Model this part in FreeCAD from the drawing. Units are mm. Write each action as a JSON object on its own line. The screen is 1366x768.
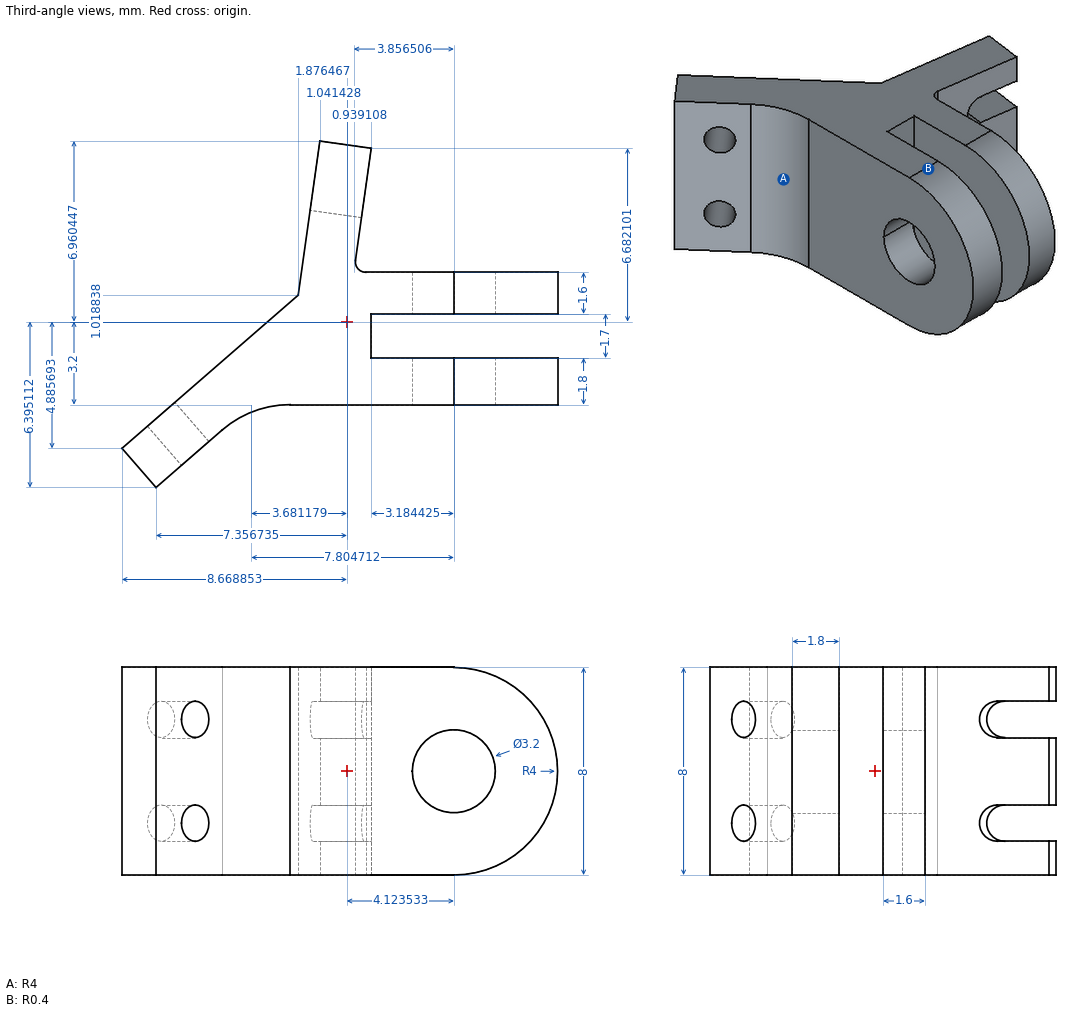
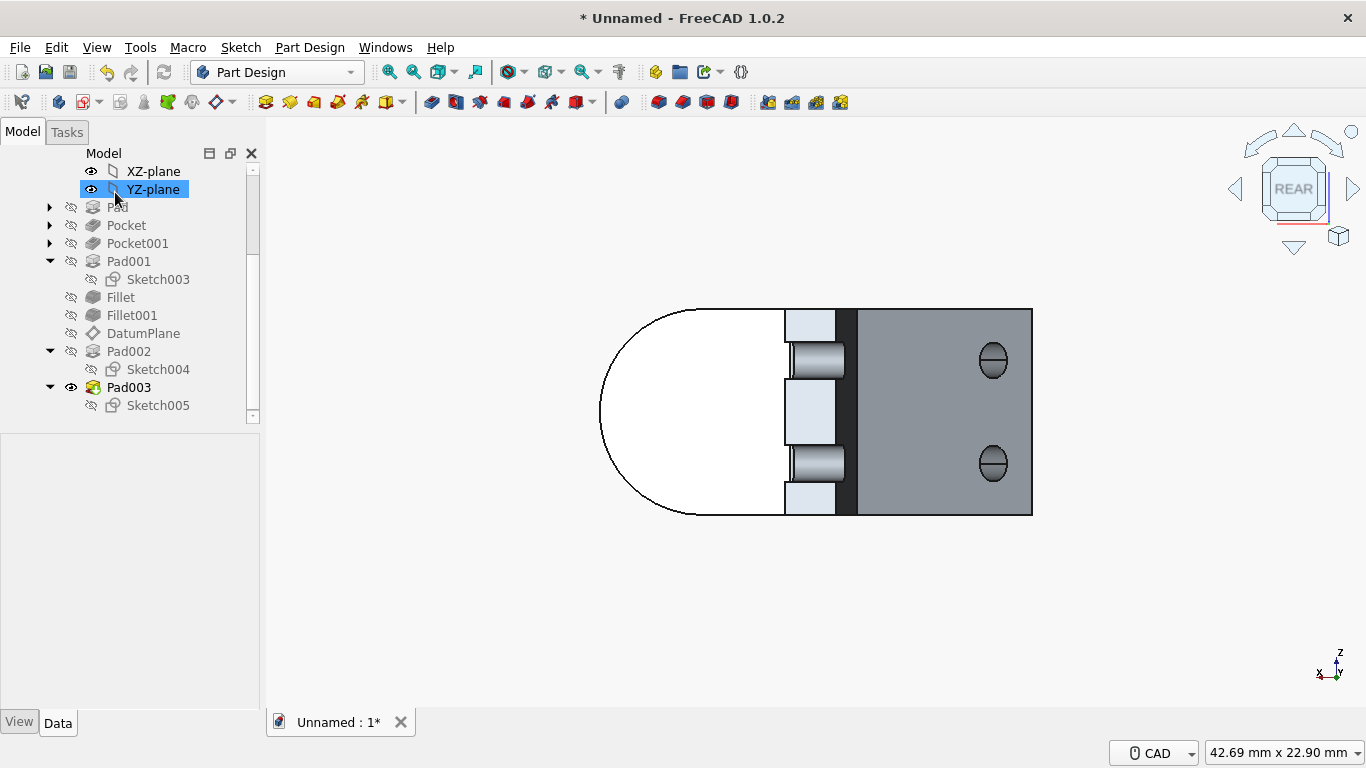
{"action": "left_click", "coordinate": [390, 72]}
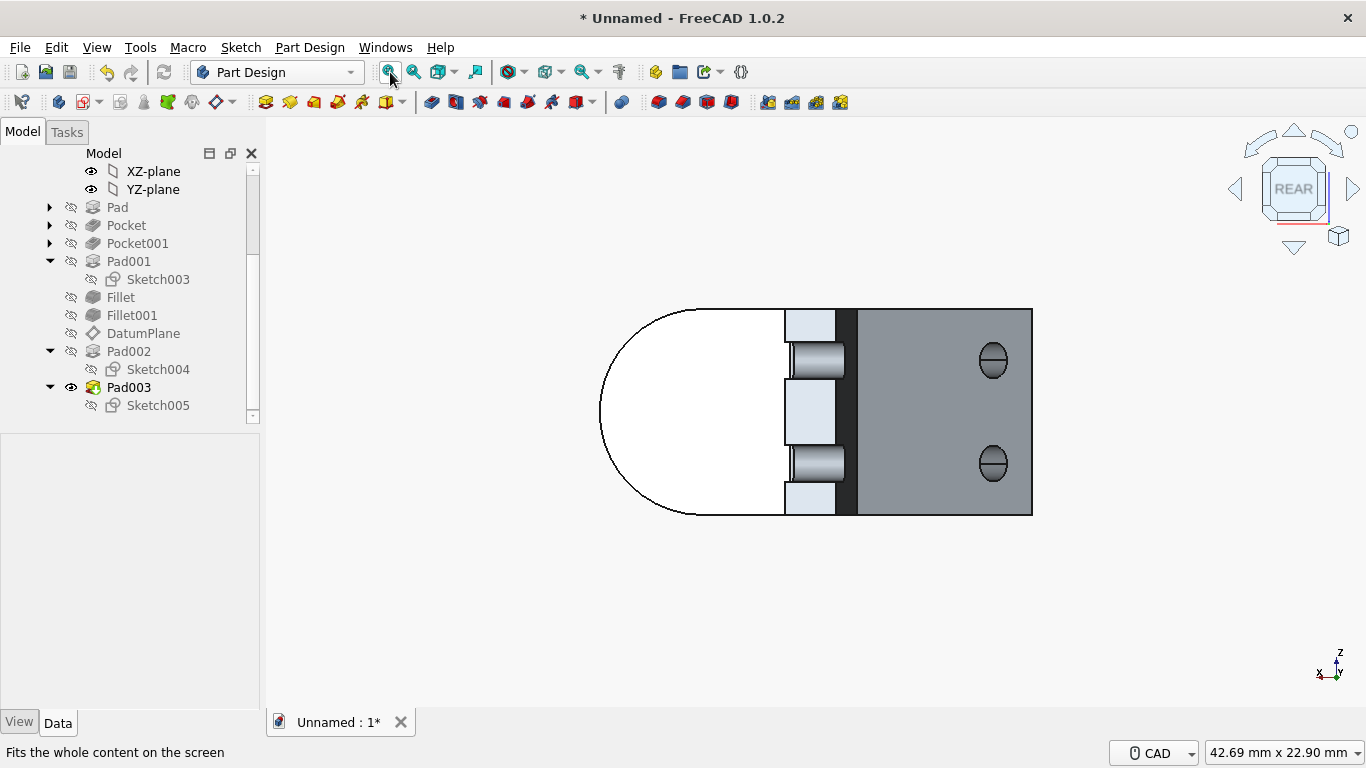
{"action": "left_click", "coordinate": [695, 411]}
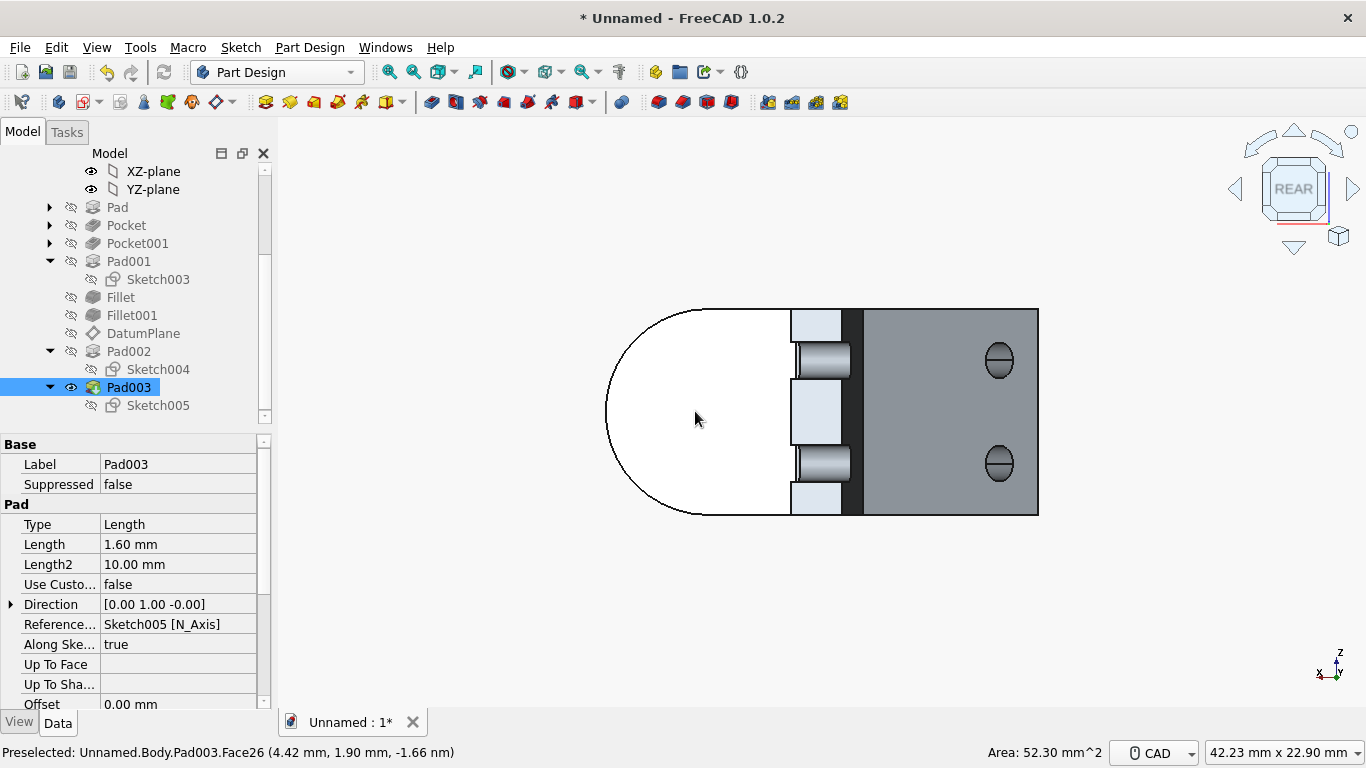
{"action": "left_click", "coordinate": [84, 102]}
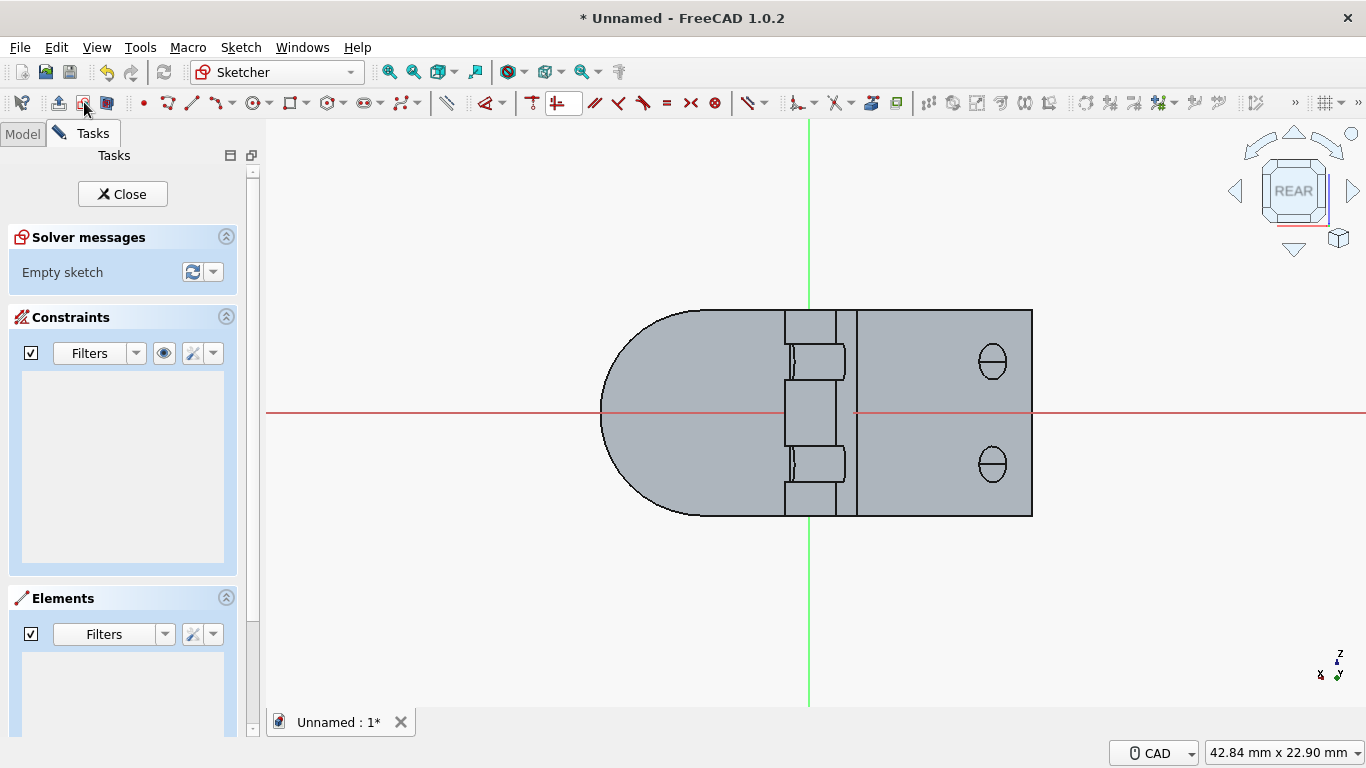
{"action": "left_click", "coordinate": [108, 104]}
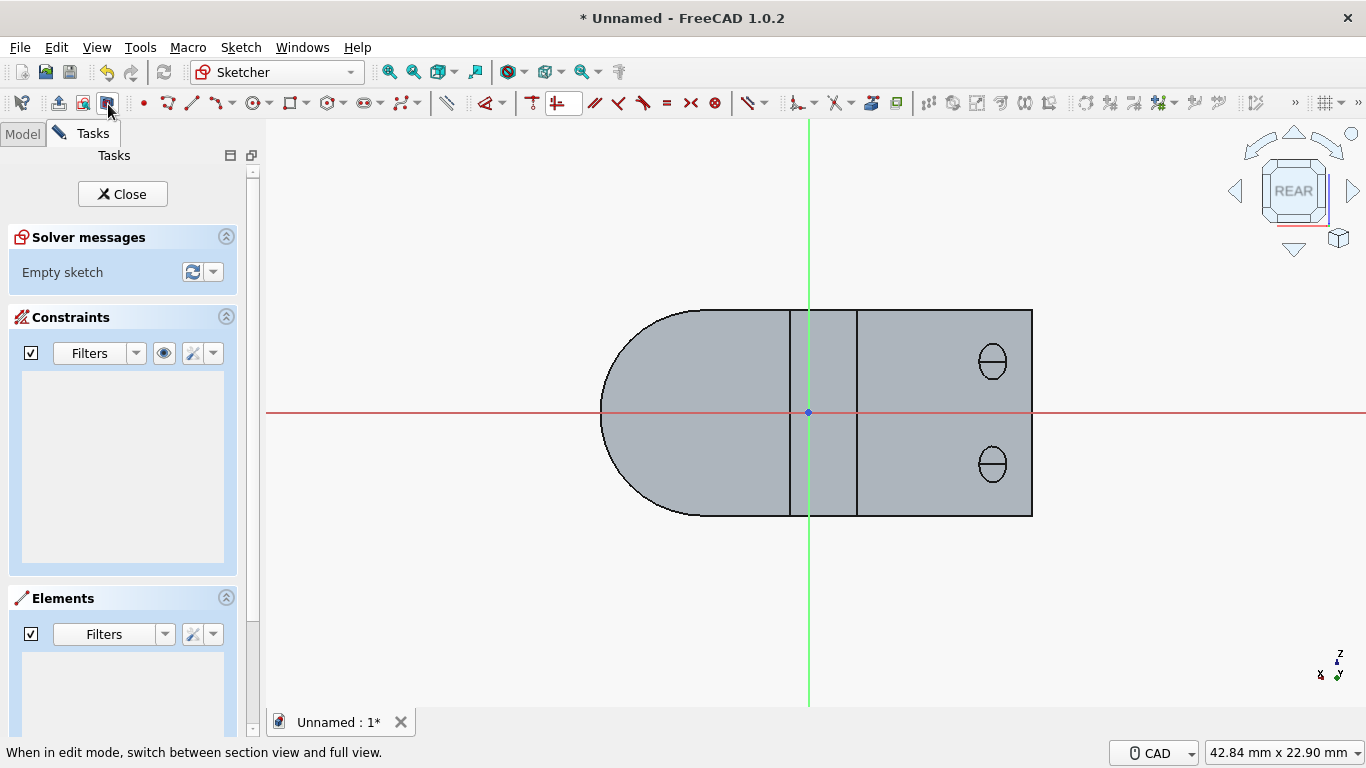
{"action": "scroll", "coordinate": [732, 413], "scroll_direction": "up", "scroll_amount": 7}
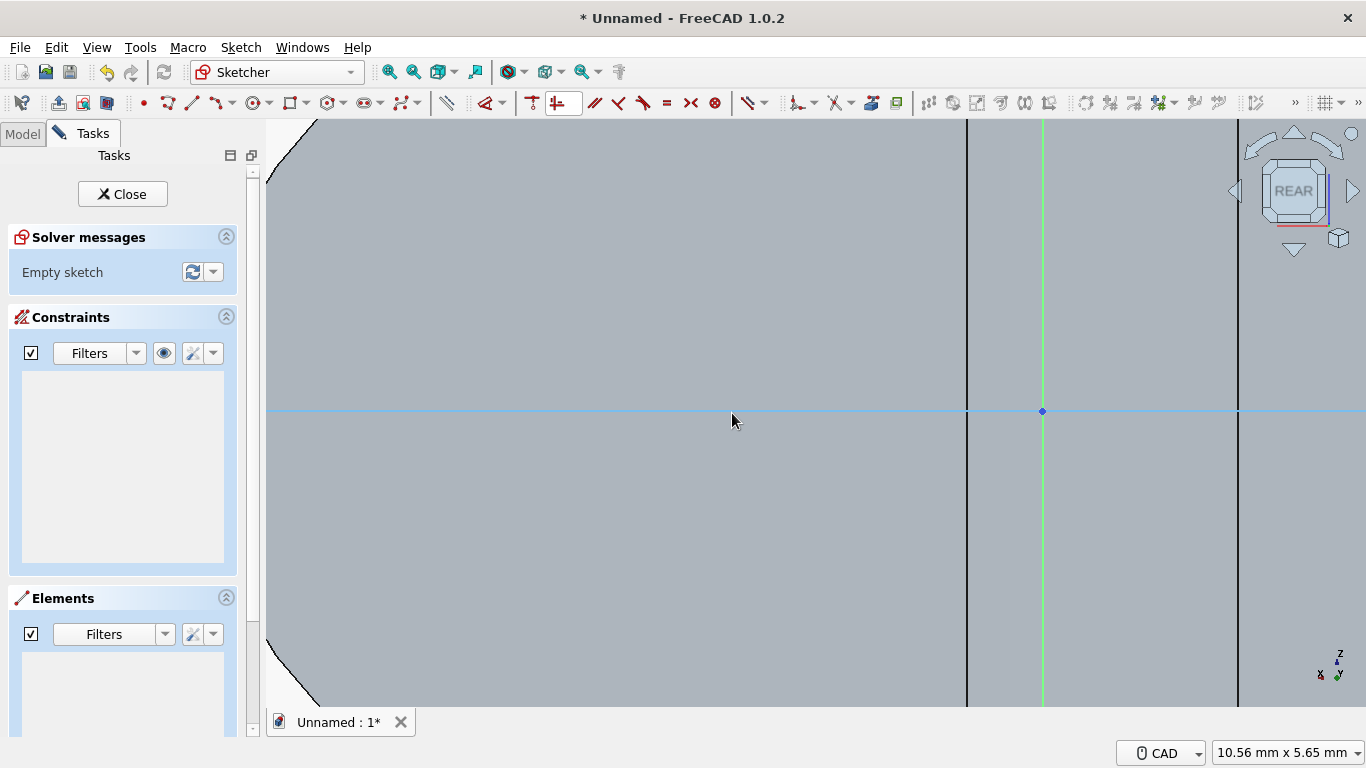
{"action": "left_click", "coordinate": [254, 104]}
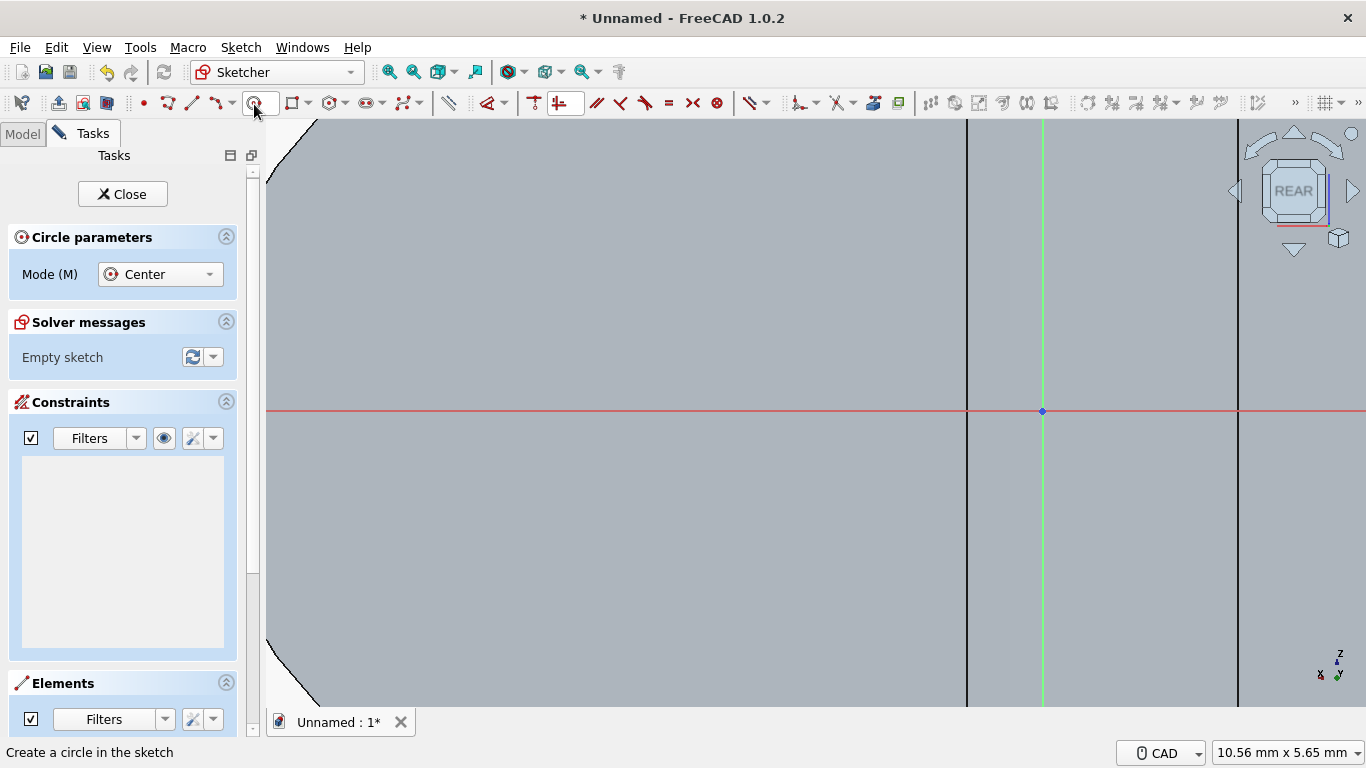
{"action": "left_click", "coordinate": [614, 411]}
{"action": "mouse_move", "coordinate": [731, 294]}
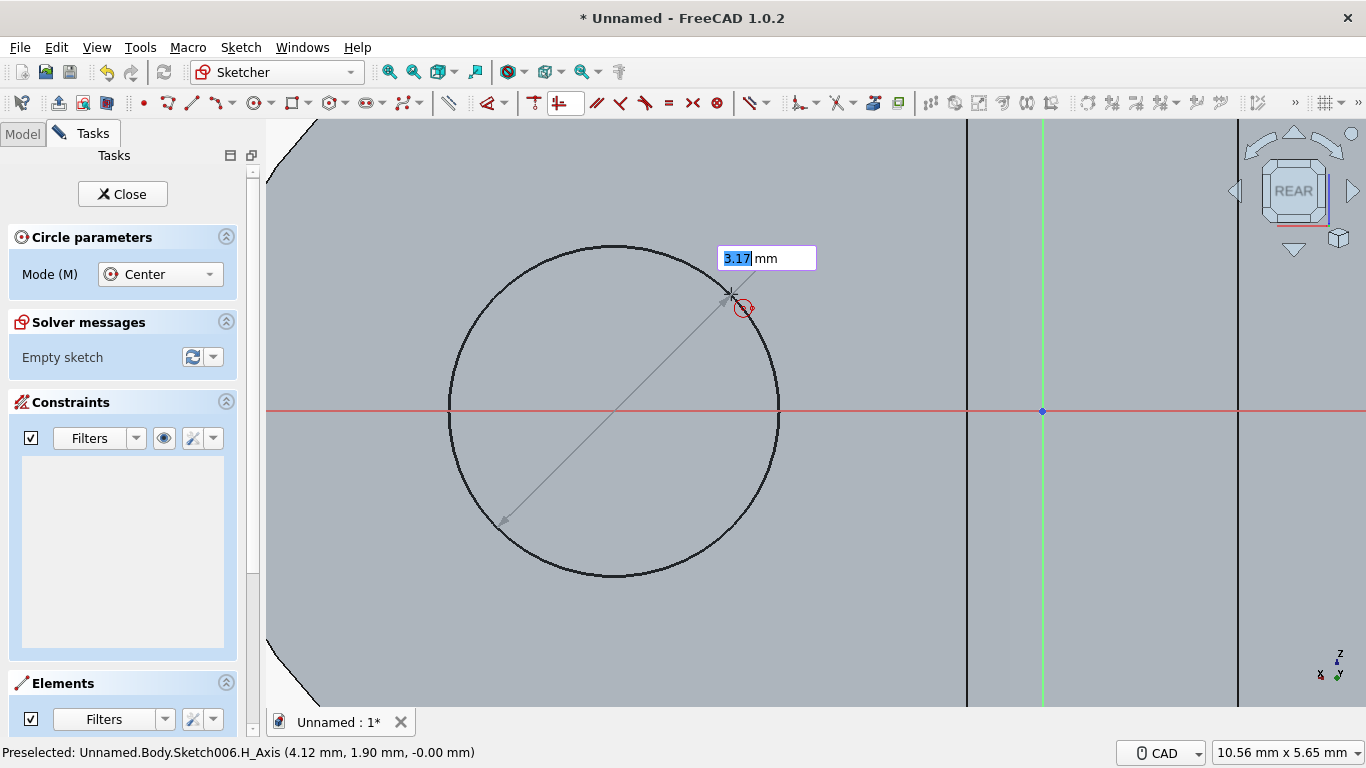
{"action": "type", "text": "3.2"}
{"action": "key", "text": "Return"}
{"action": "key", "text": "Escape"}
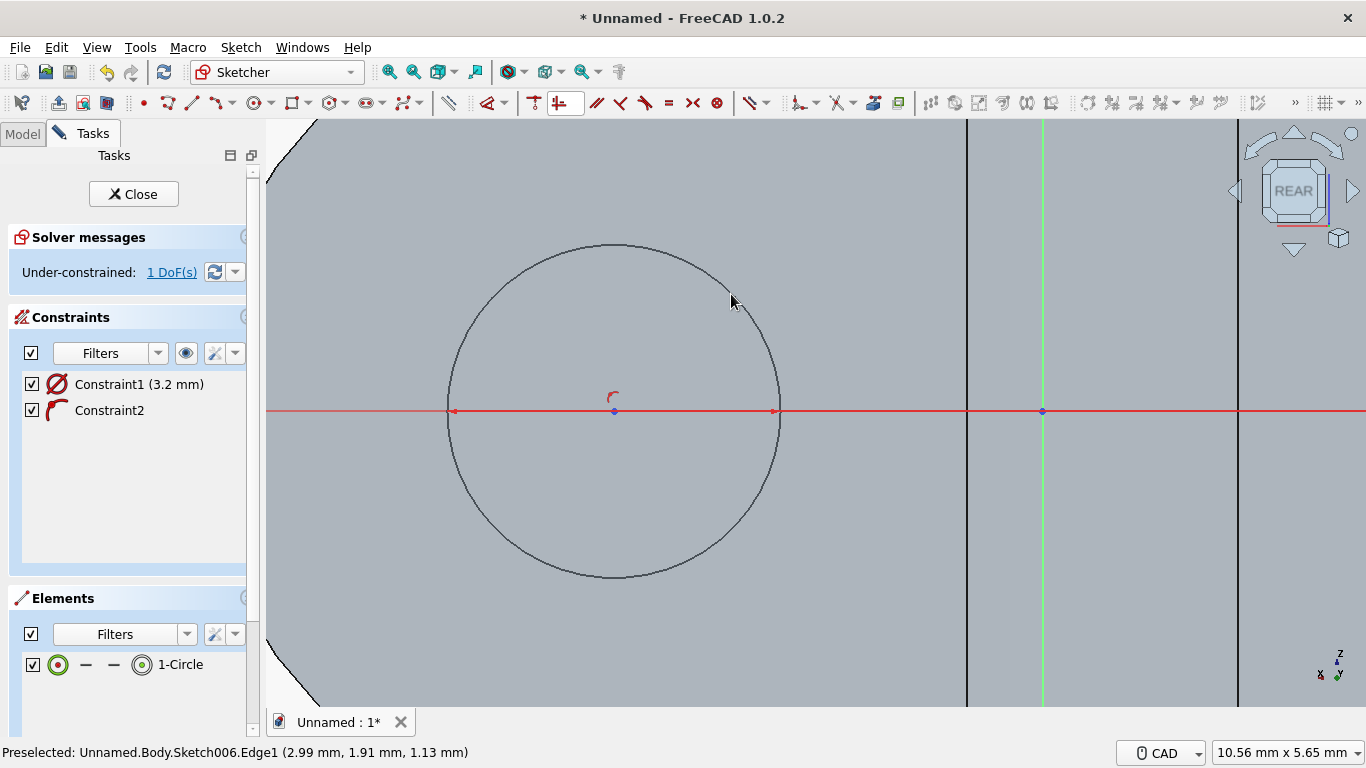
{"action": "left_click", "coordinate": [488, 104]}